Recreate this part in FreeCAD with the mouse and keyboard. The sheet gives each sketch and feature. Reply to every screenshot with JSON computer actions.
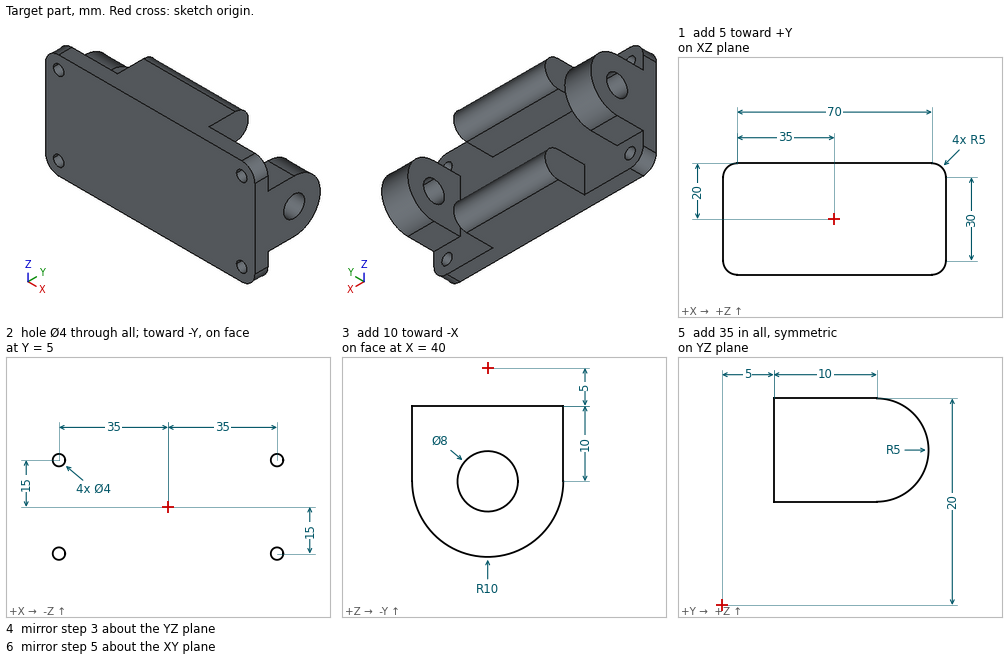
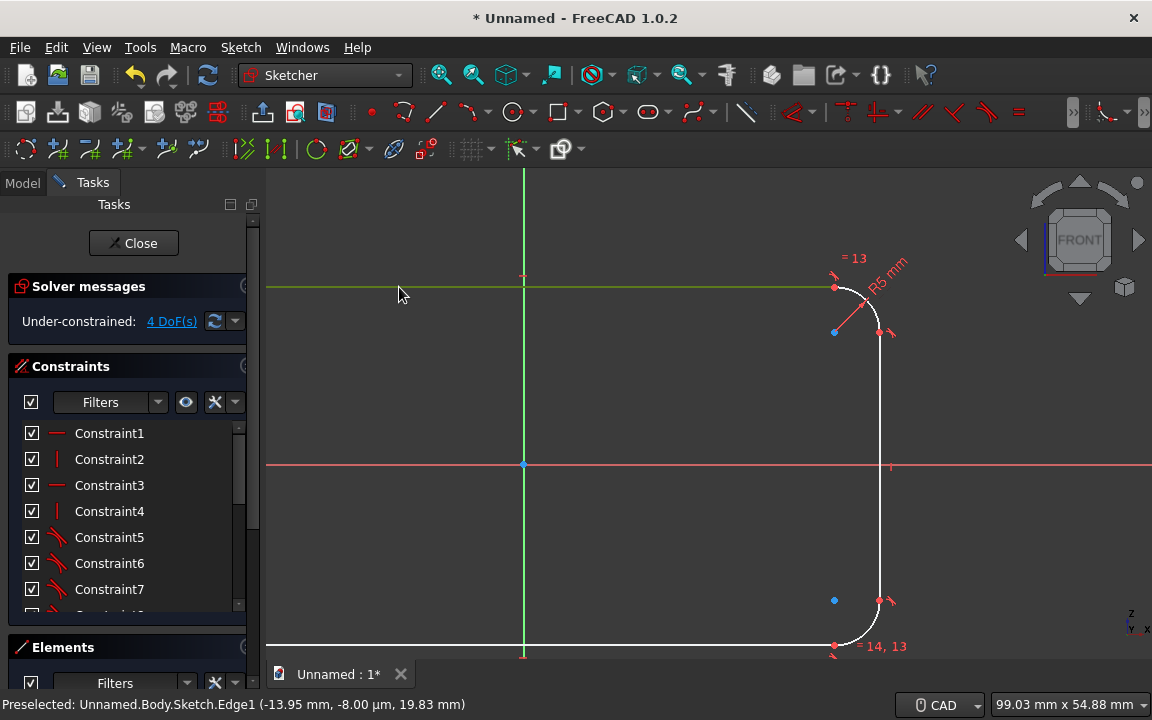
{"action": "left_click", "coordinate": [814, 112]}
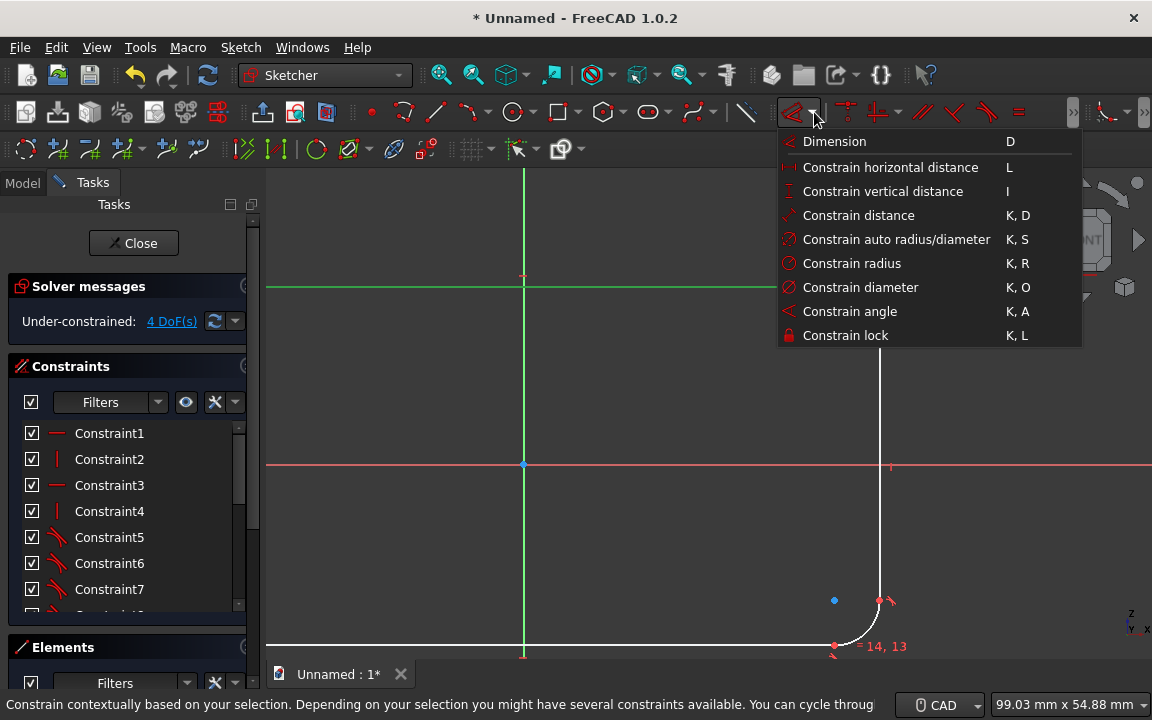
{"action": "left_click", "coordinate": [930, 167]}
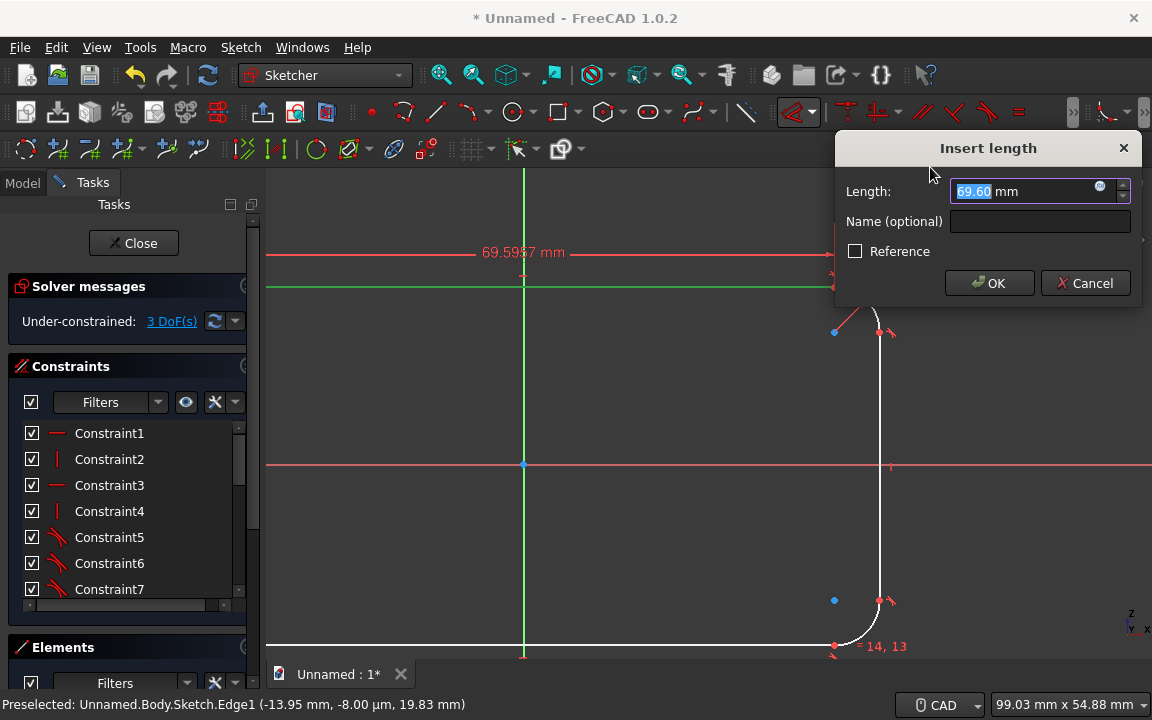
{"action": "type", "text": "70"}
{"action": "key", "text": "Return"}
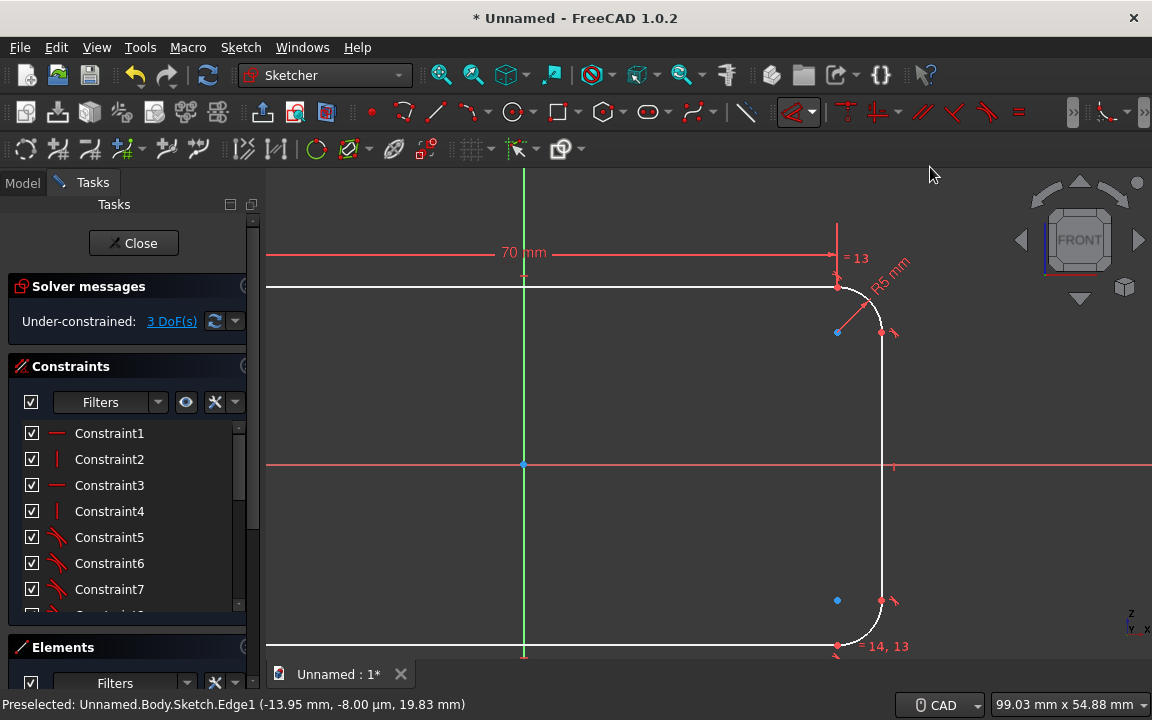
{"action": "left_click", "coordinate": [882, 413]}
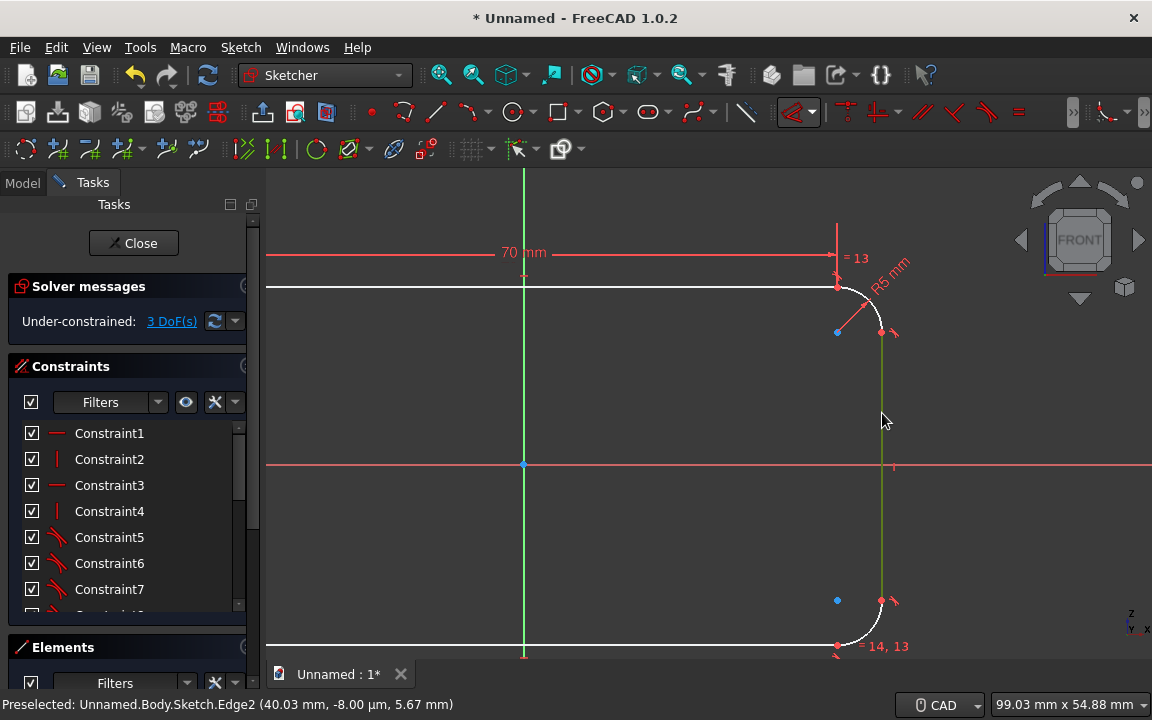
{"action": "left_click", "coordinate": [814, 112]}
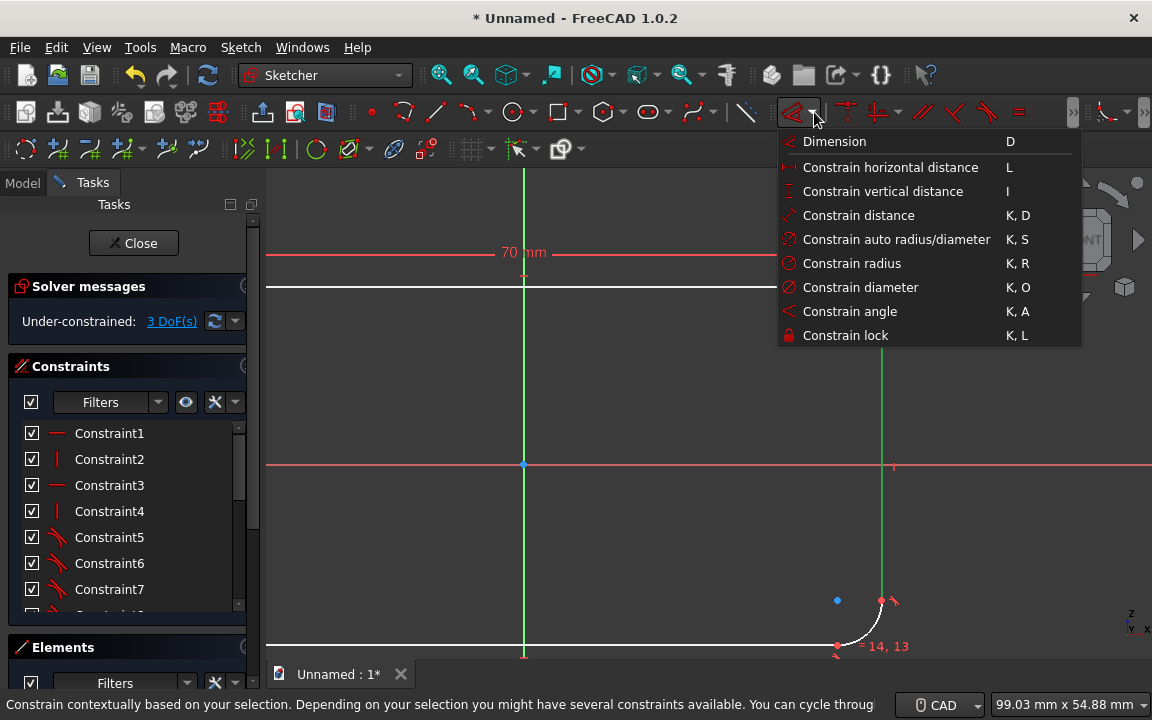
{"action": "left_click", "coordinate": [930, 191]}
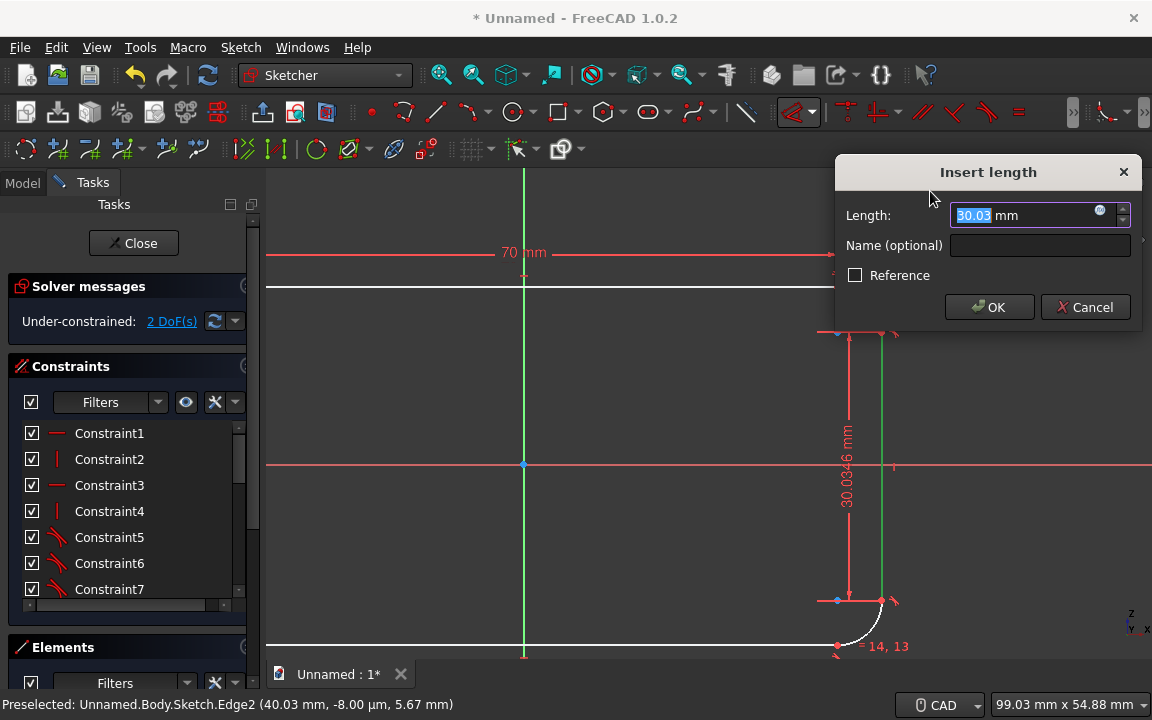
{"action": "type", "text": "30"}
{"action": "key", "text": "Return"}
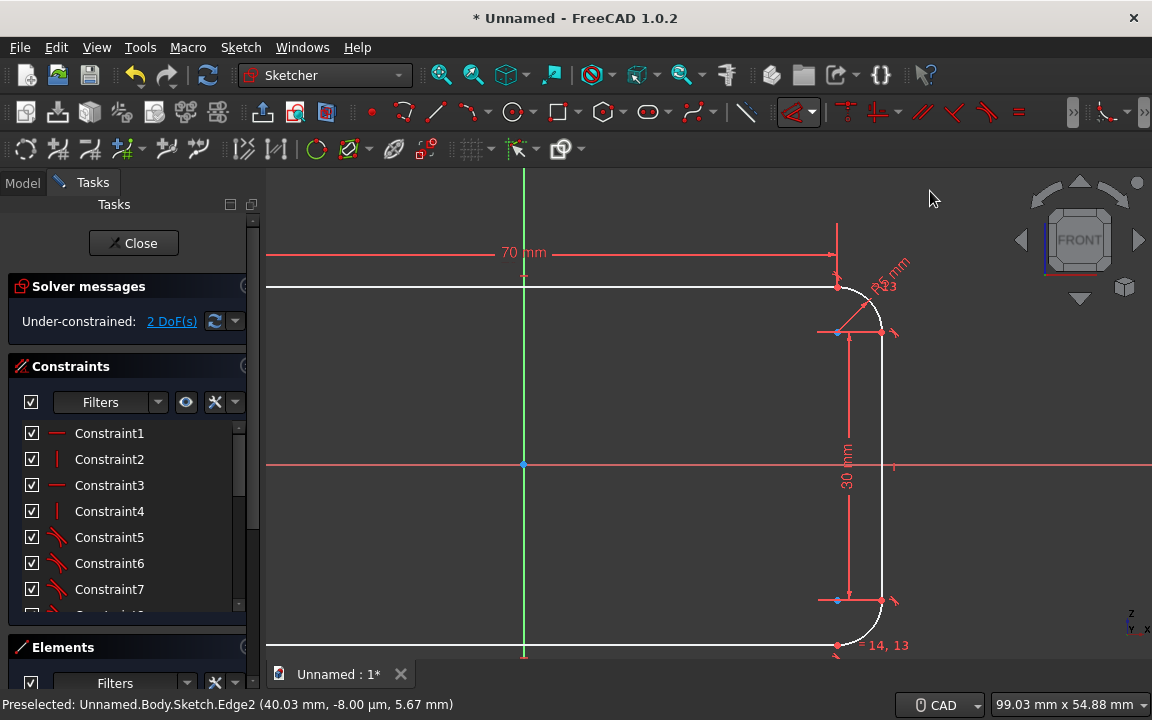
{"action": "scroll", "coordinate": [878, 309], "scroll_direction": "down", "scroll_amount": 2}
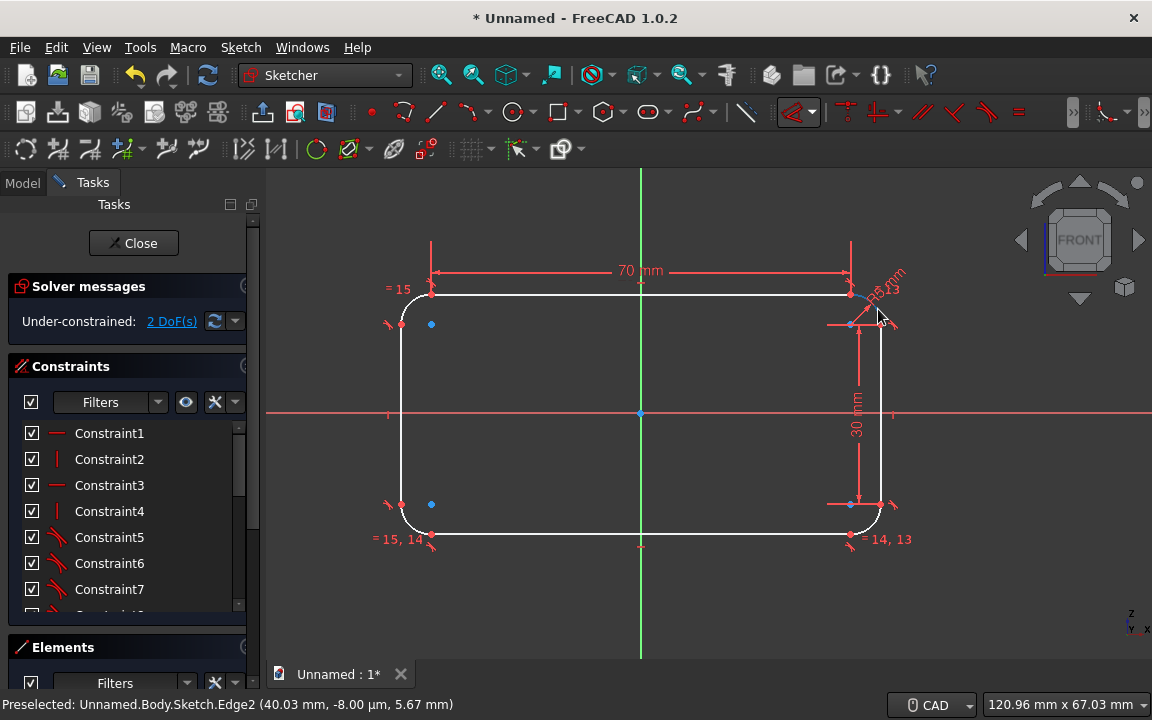
{"action": "left_click", "coordinate": [431, 295]}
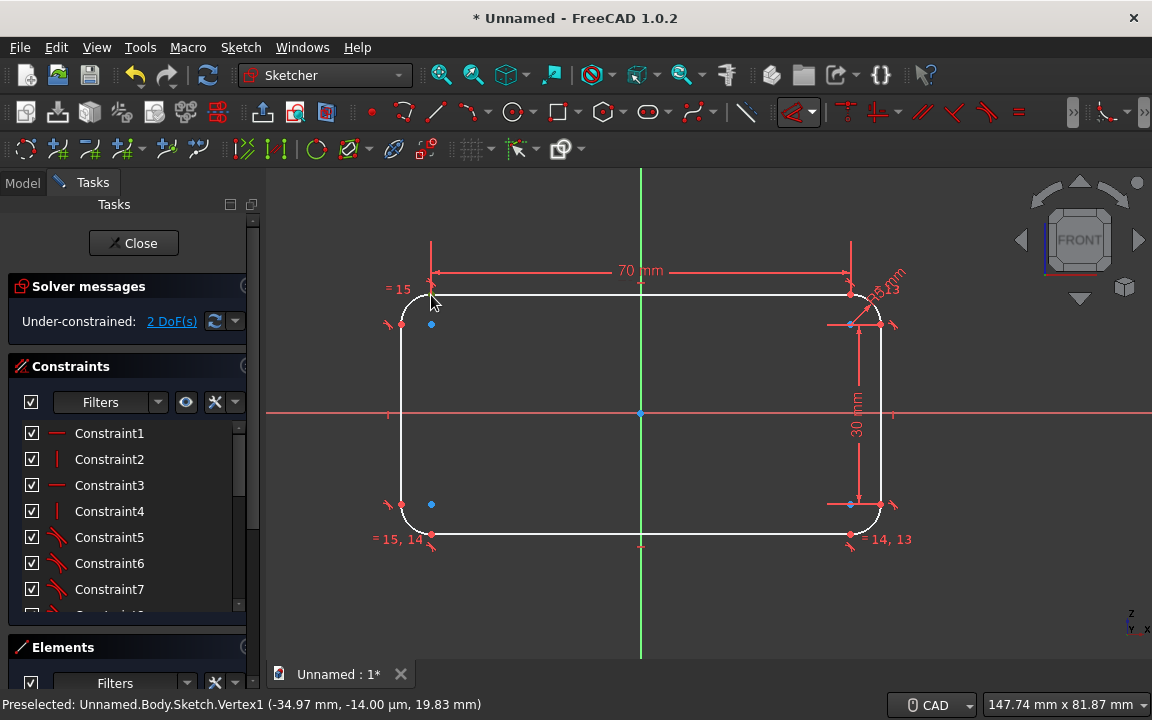
{"action": "key", "text": "l"}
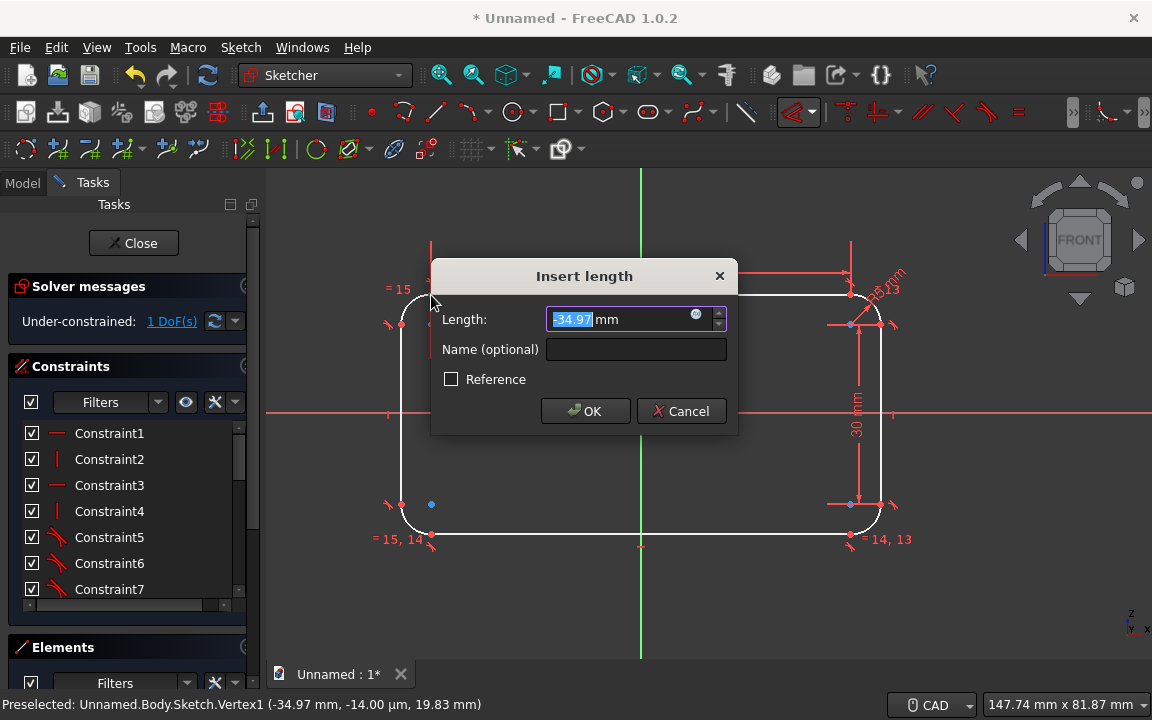
{"action": "type", "text": "-35"}
{"action": "key", "text": "Return"}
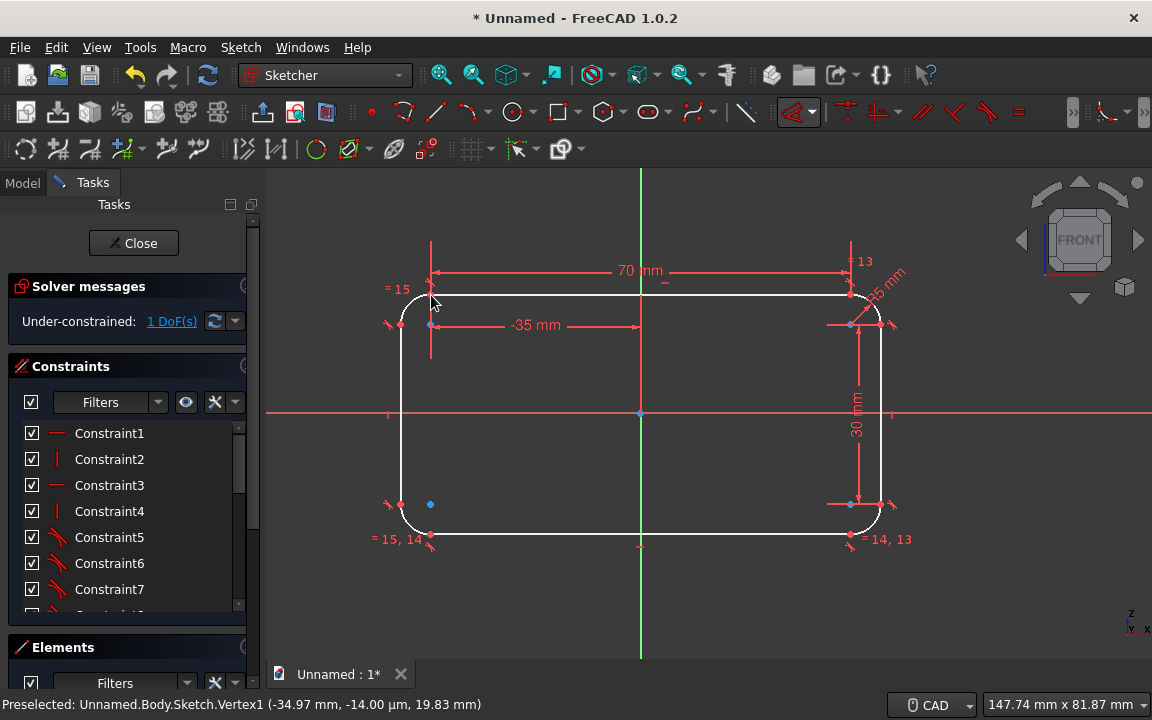
{"action": "left_click", "coordinate": [431, 295]}